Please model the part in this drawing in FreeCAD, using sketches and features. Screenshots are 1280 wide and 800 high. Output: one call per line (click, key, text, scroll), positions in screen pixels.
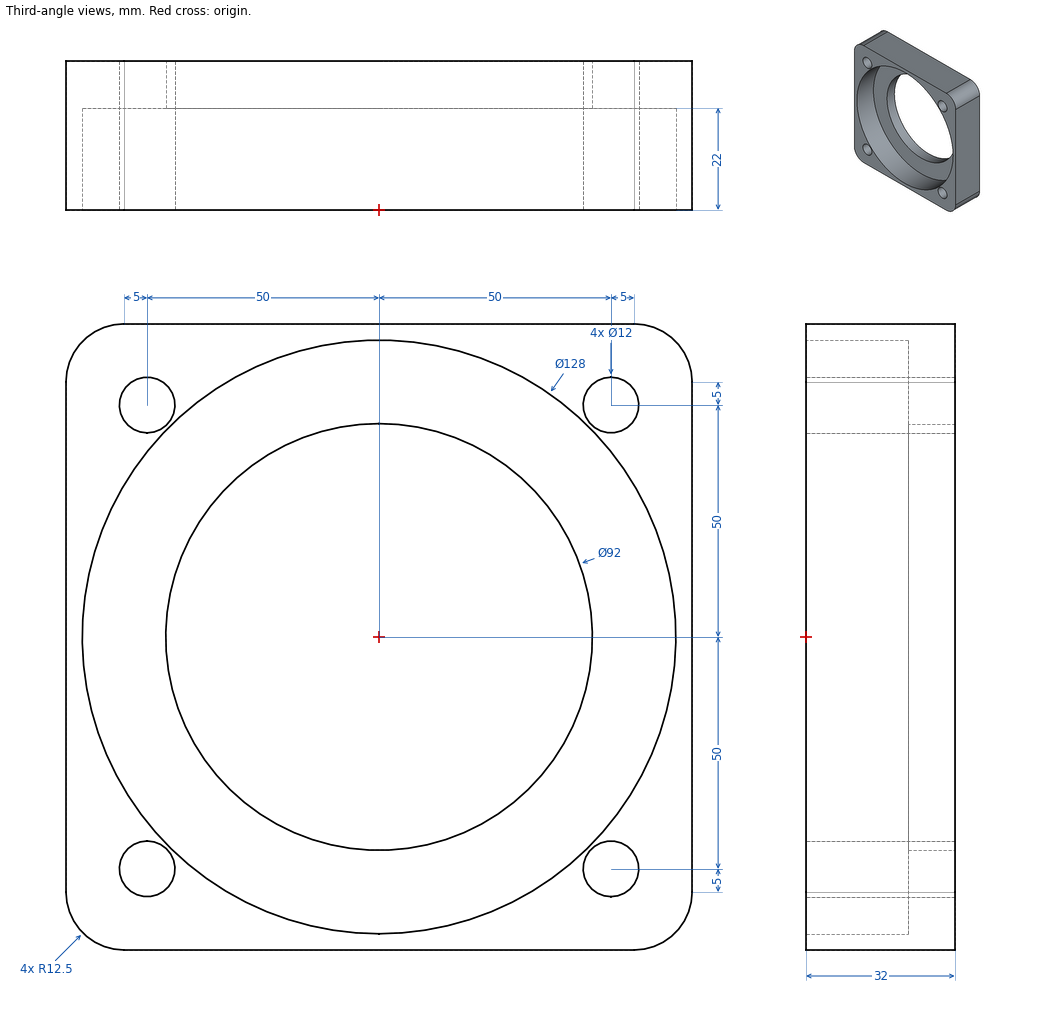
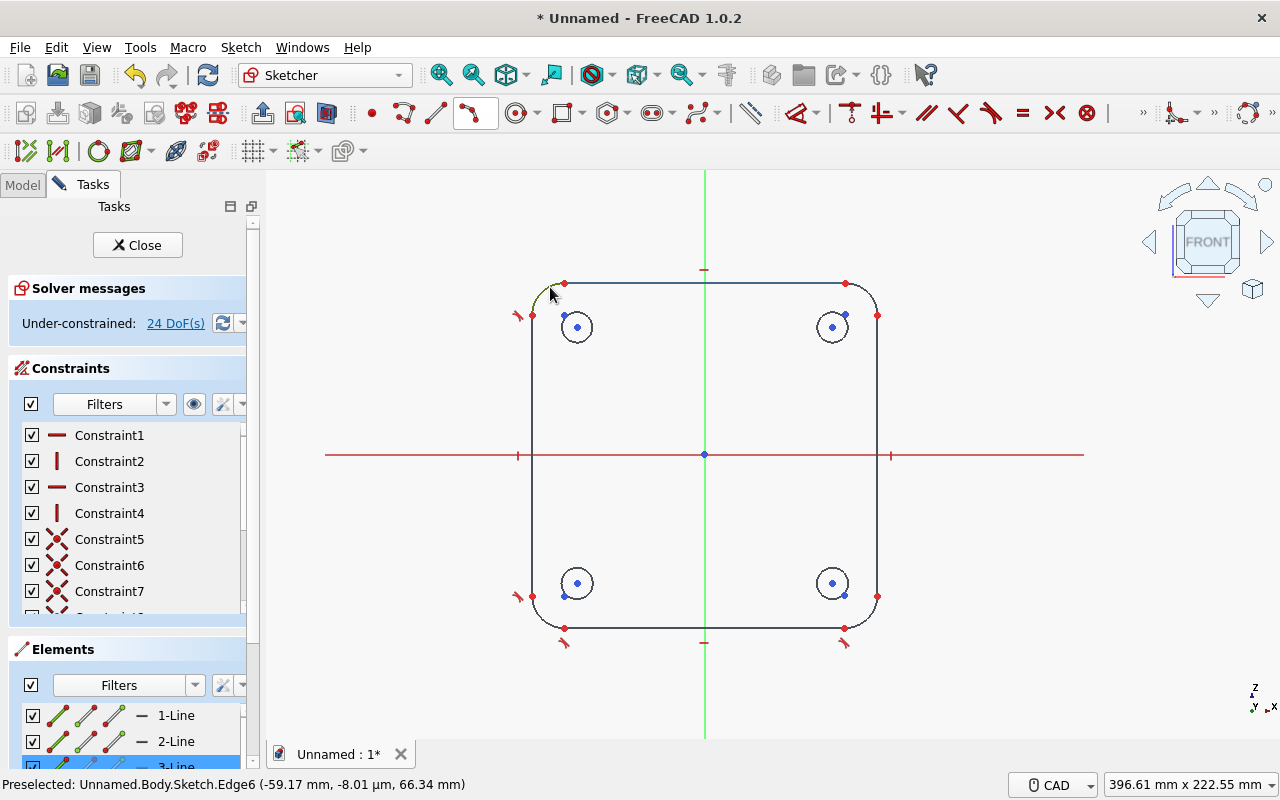
click(992, 114)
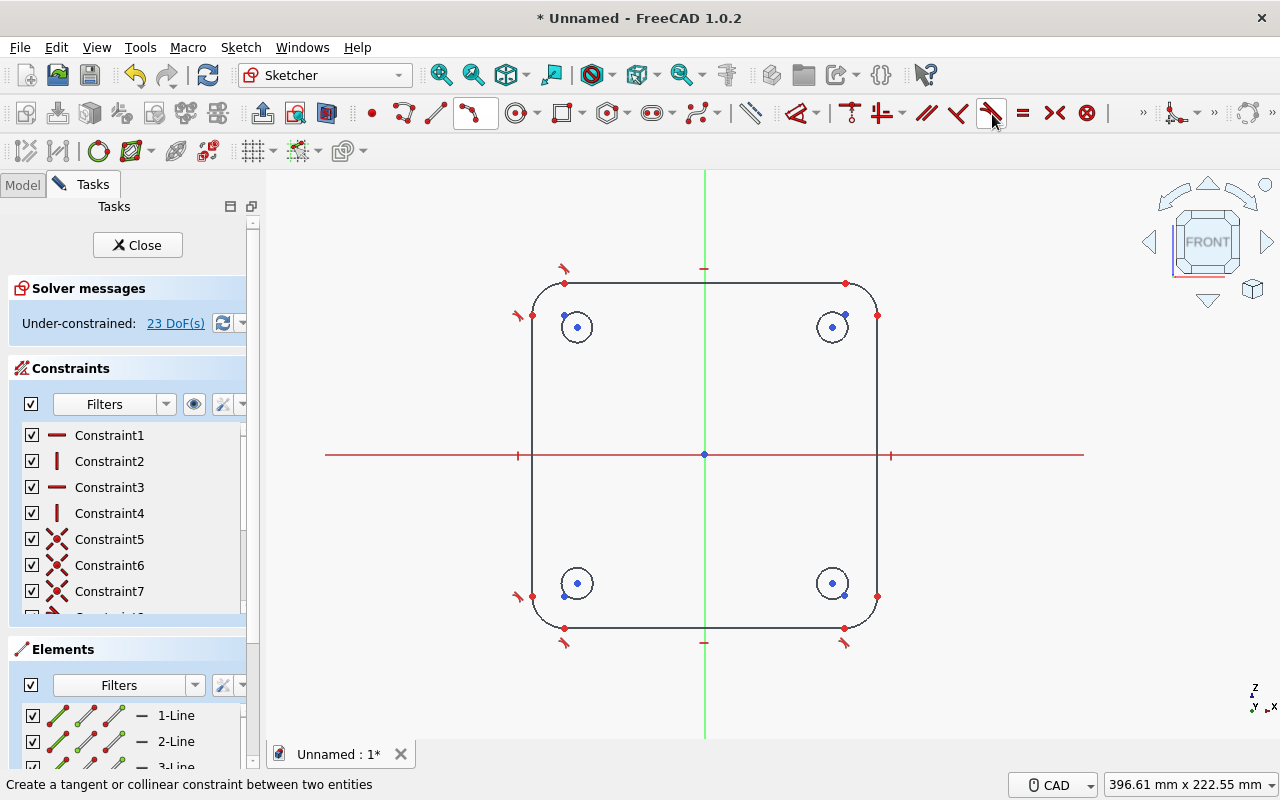
click(649, 283)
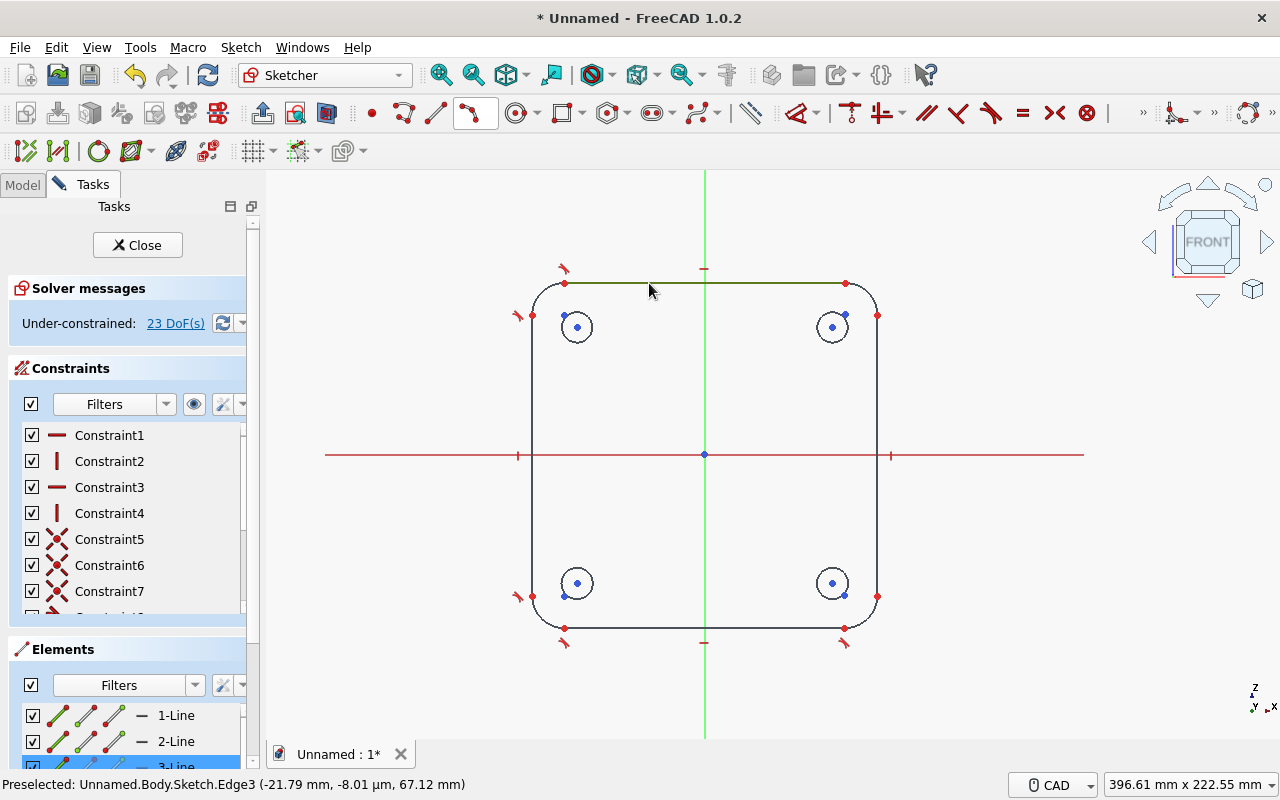
click(874, 301)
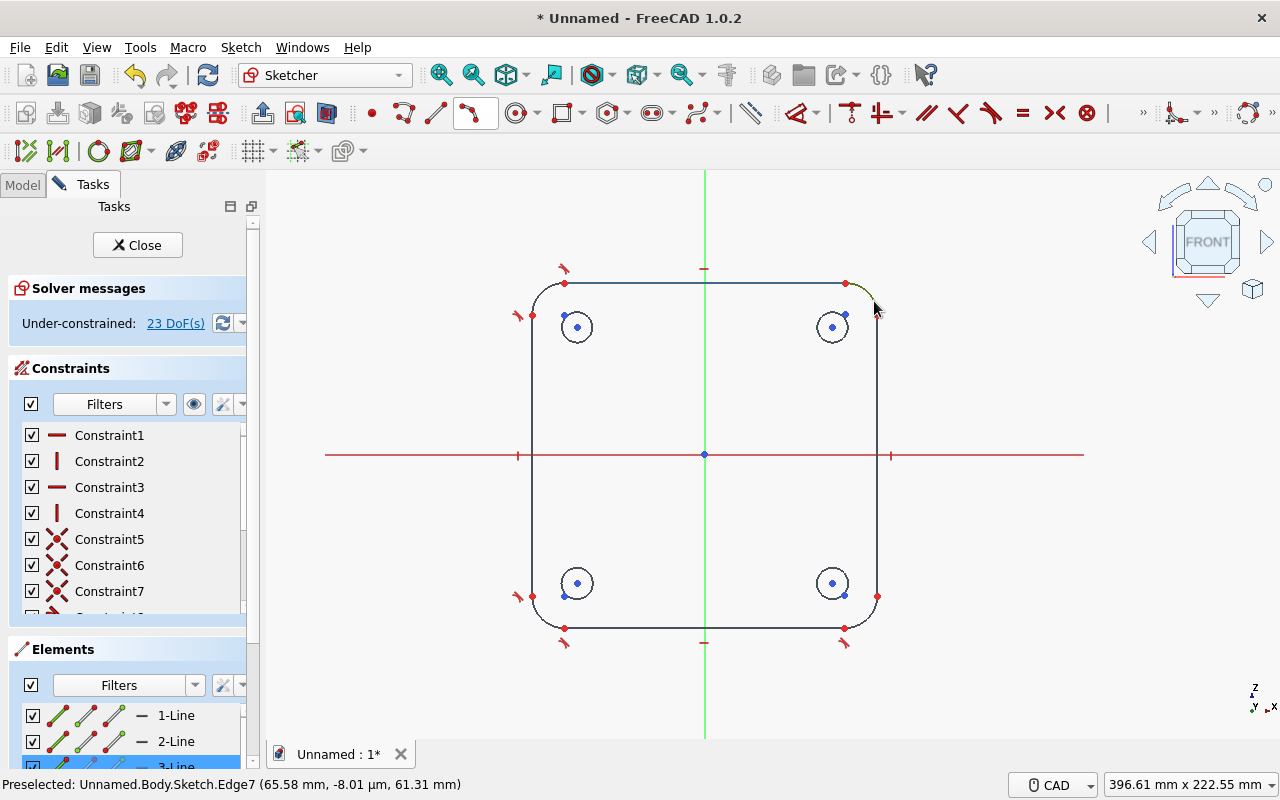
click(992, 114)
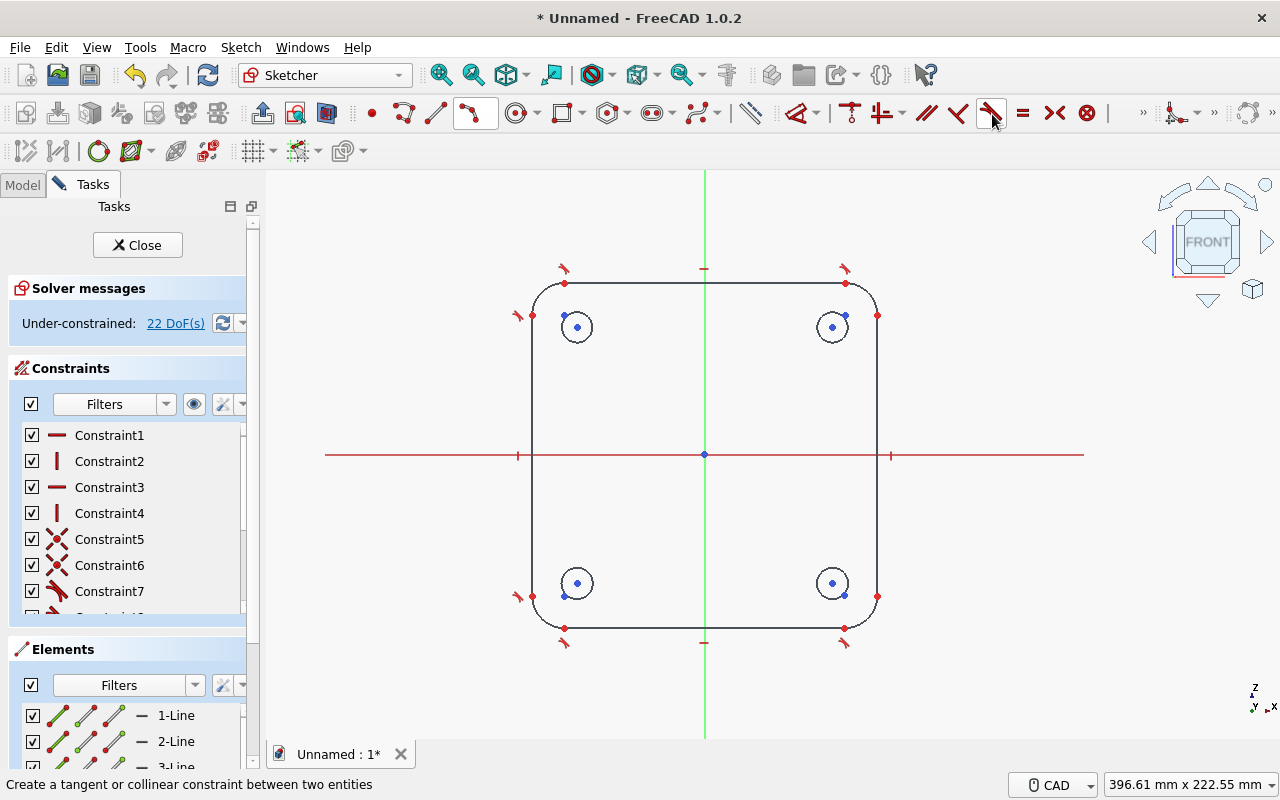
click(877, 399)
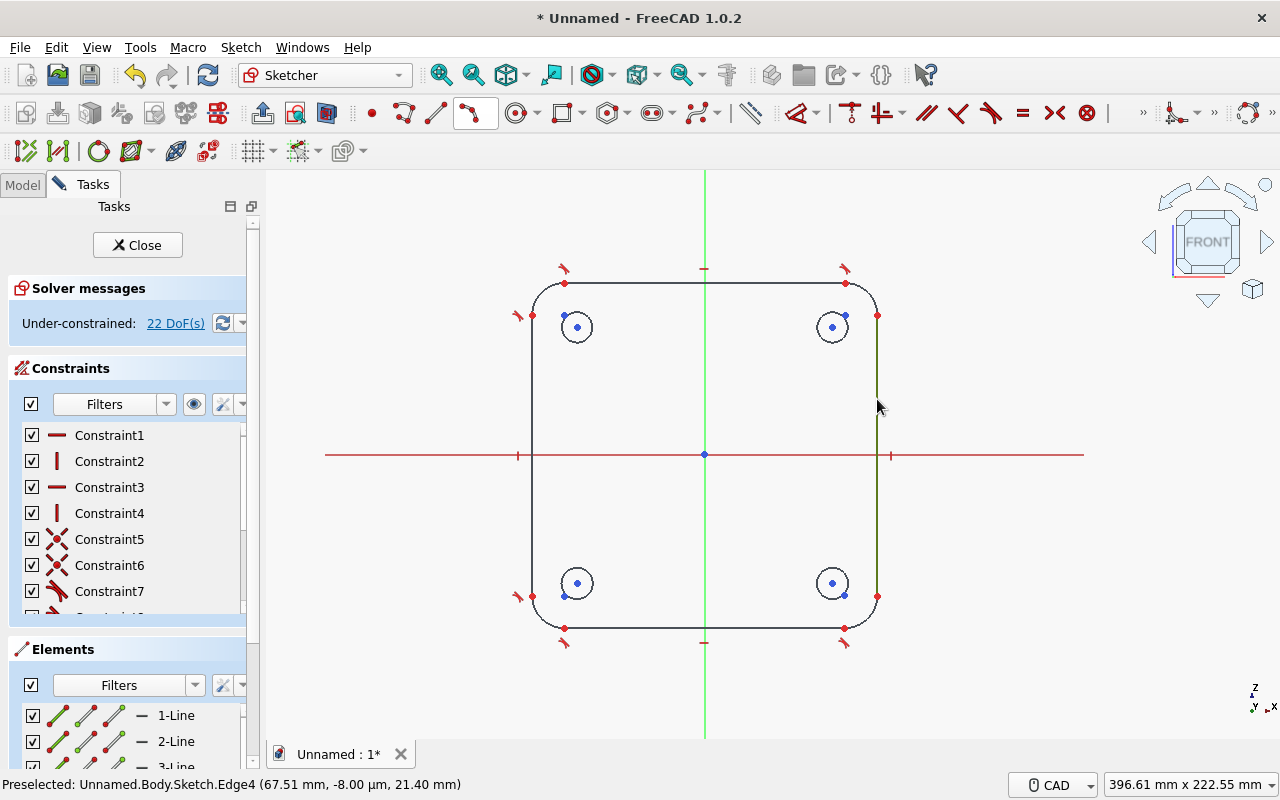
click(874, 301)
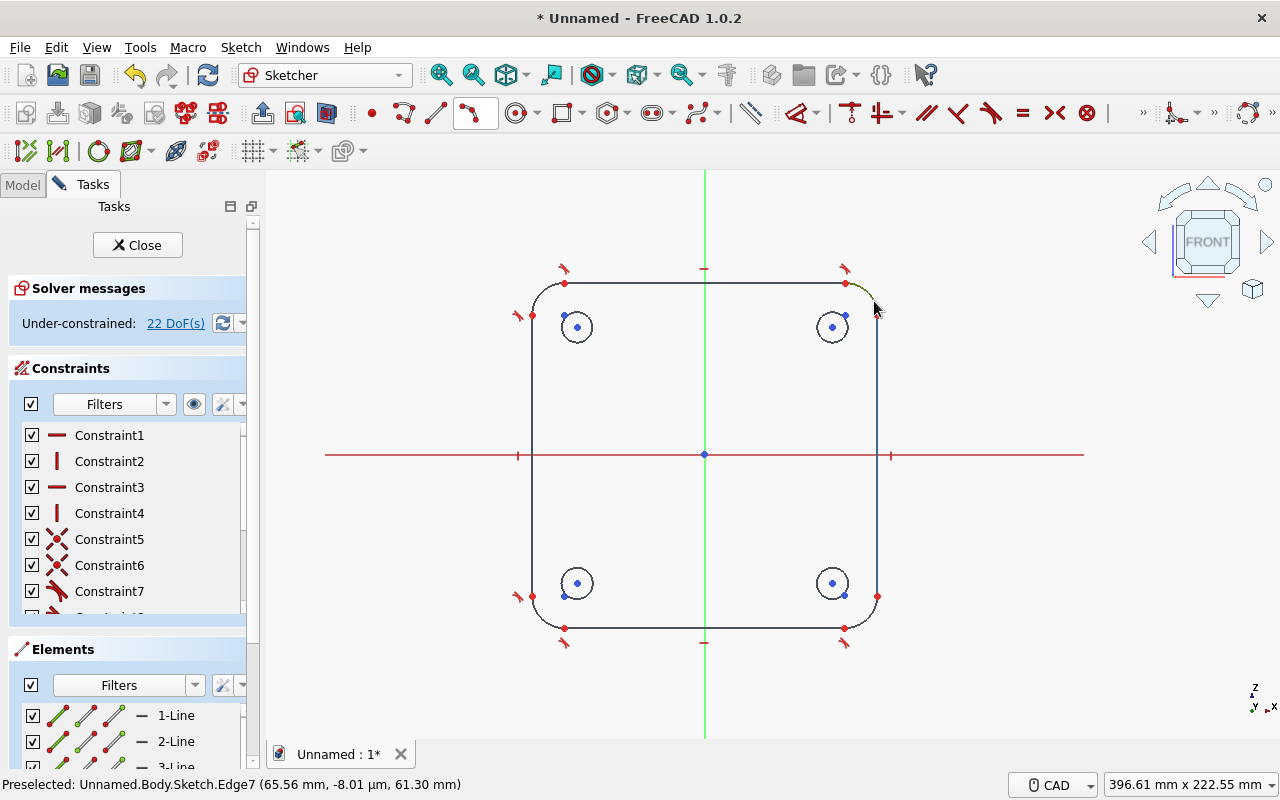
click(992, 114)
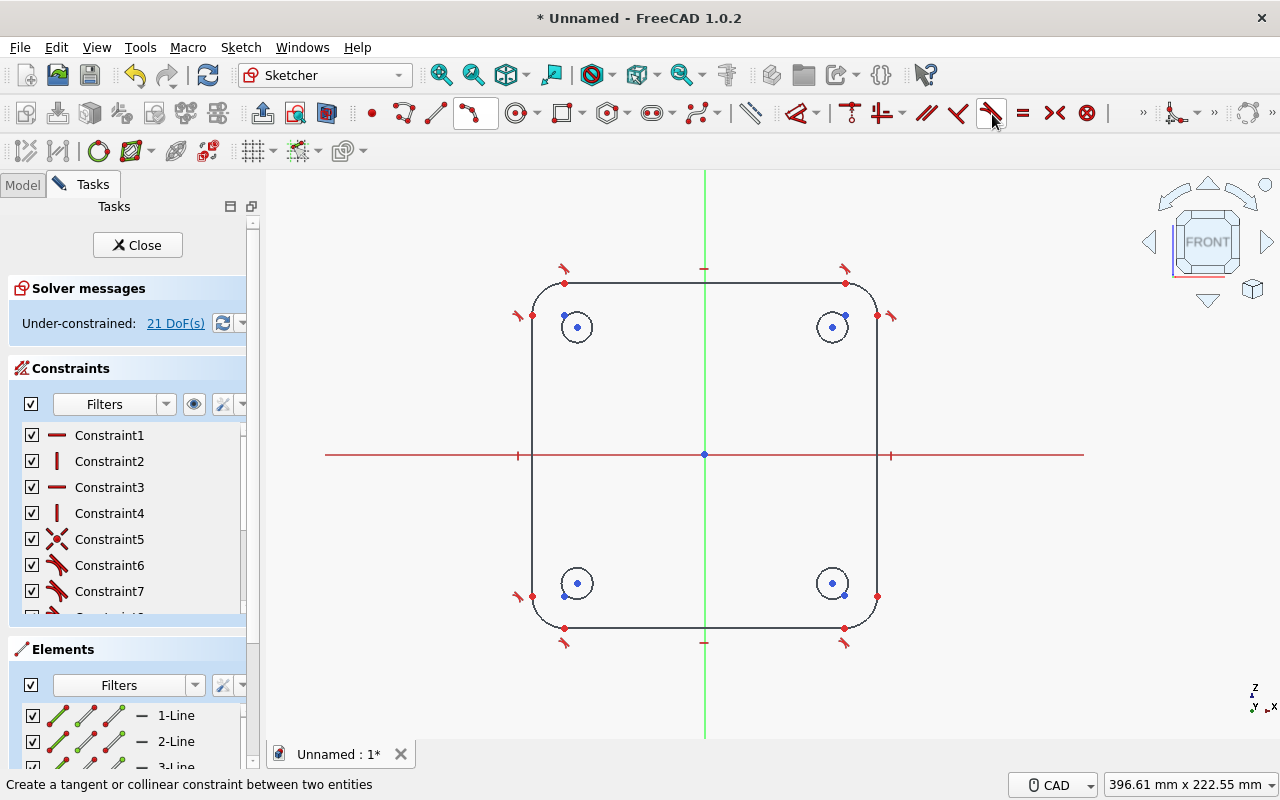
click(877, 399)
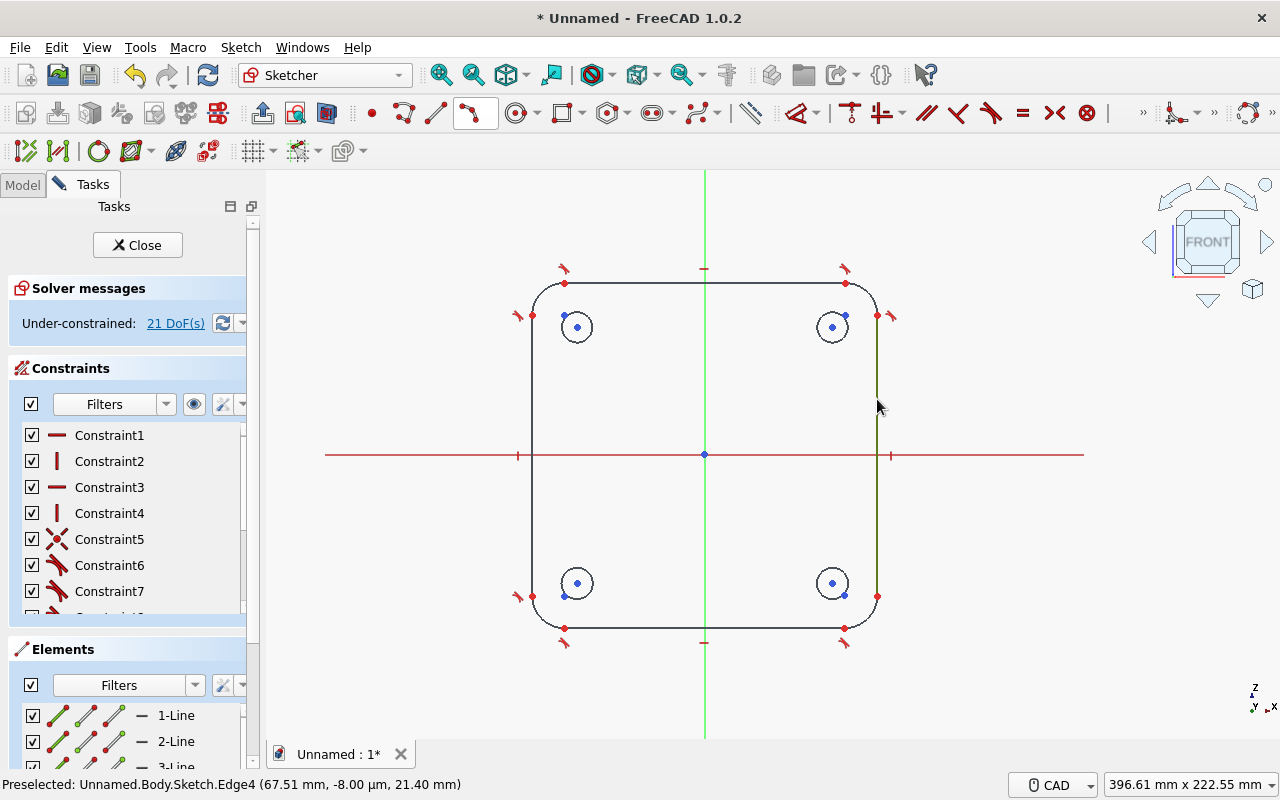
click(859, 625)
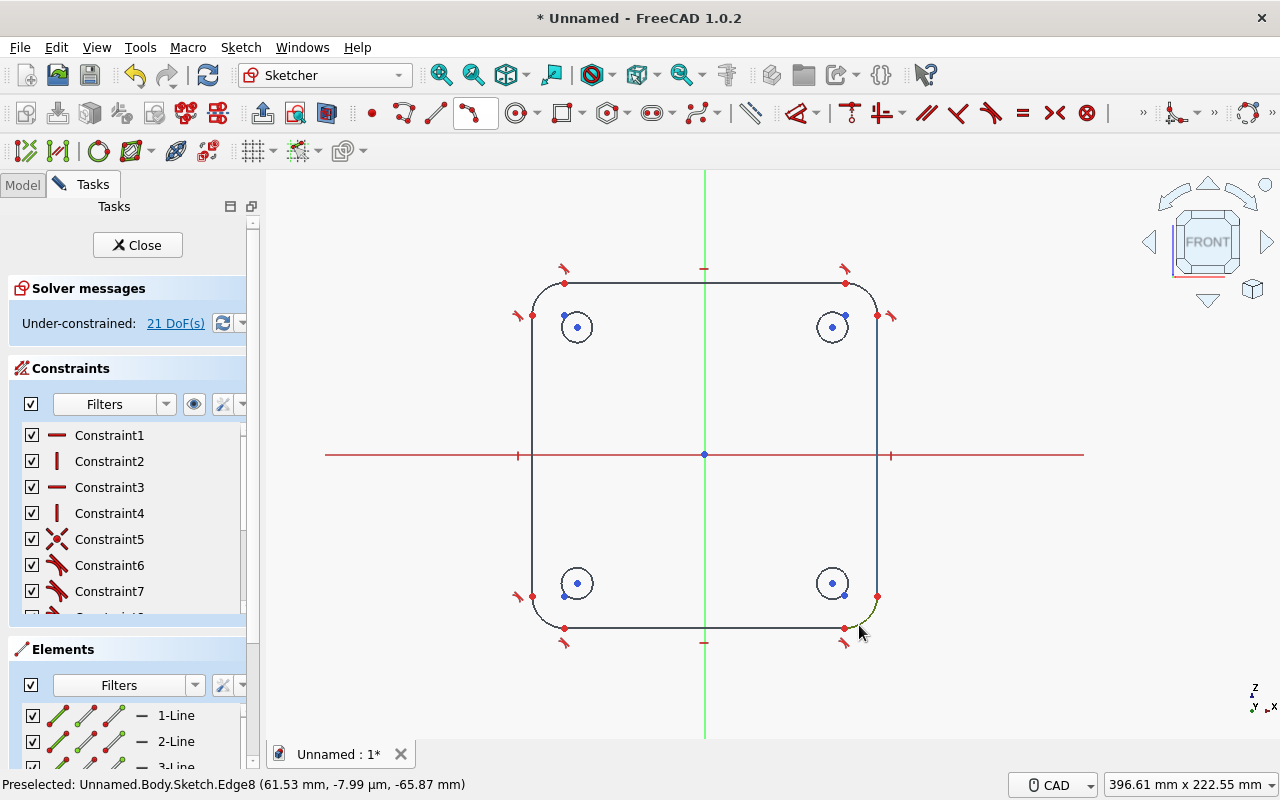
click(992, 114)